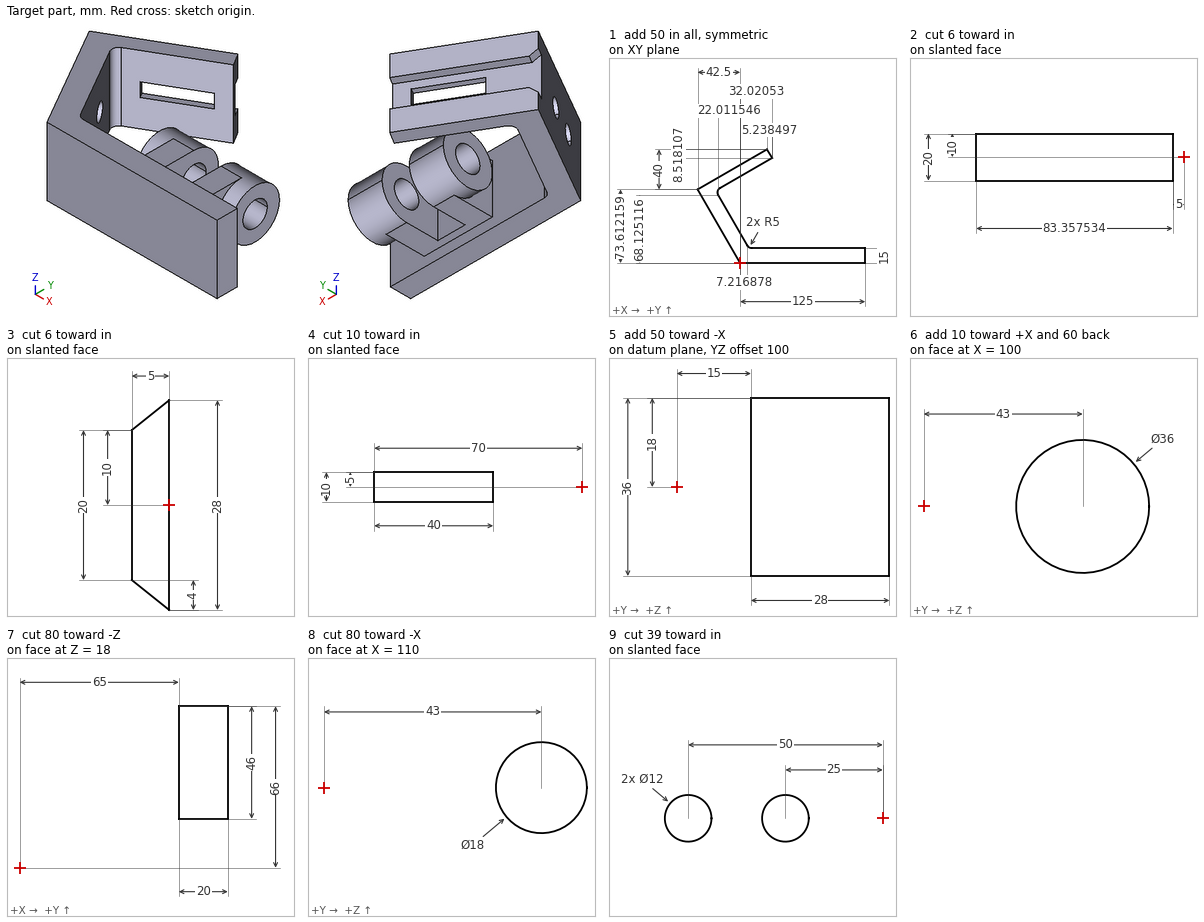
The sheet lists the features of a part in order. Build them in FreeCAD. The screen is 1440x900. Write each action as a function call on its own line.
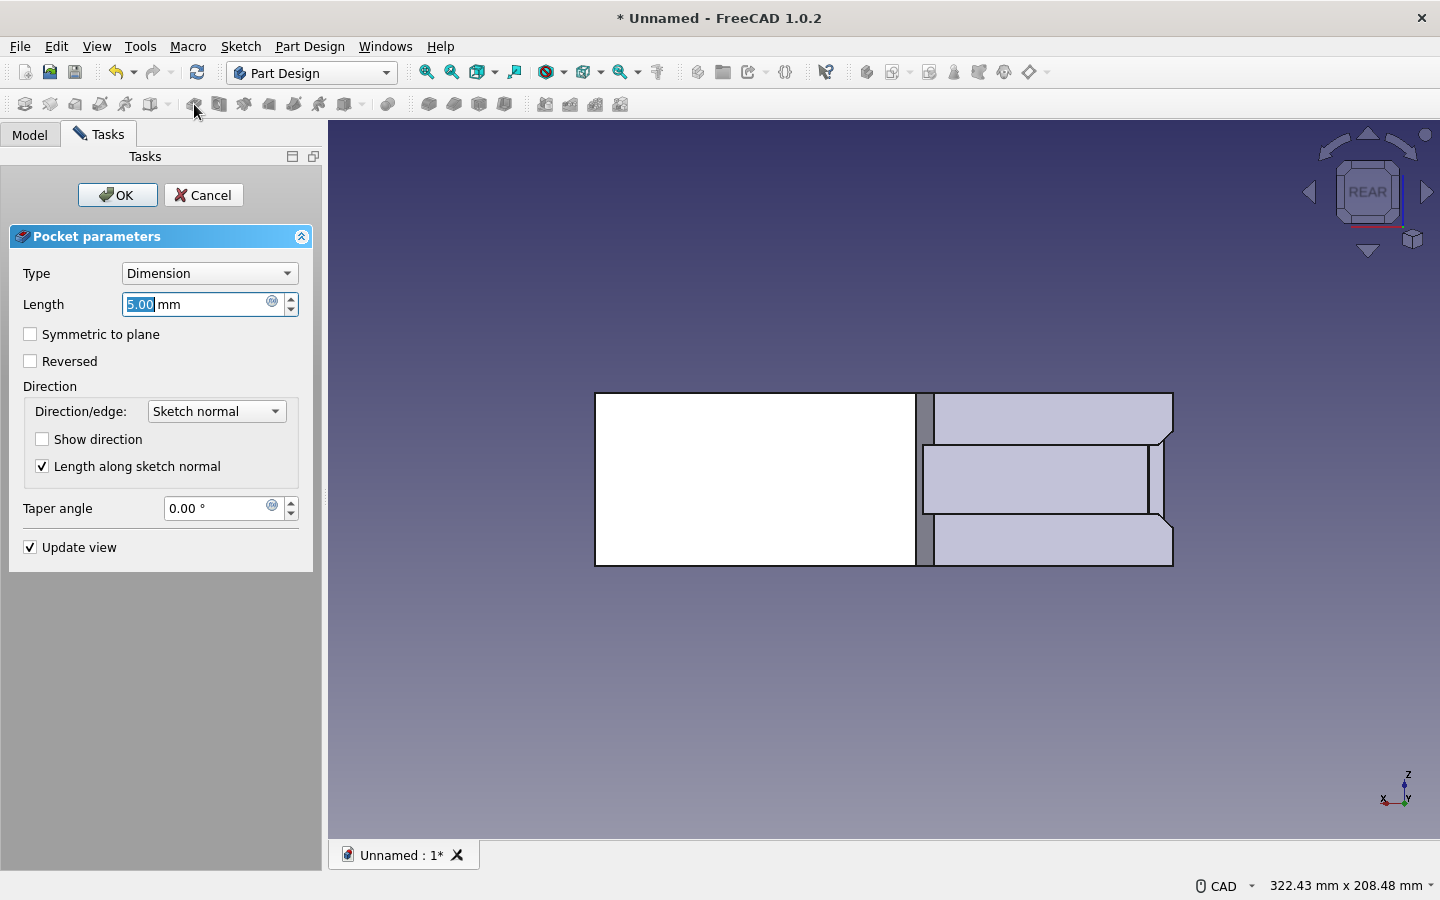
text(6)
key(Tab)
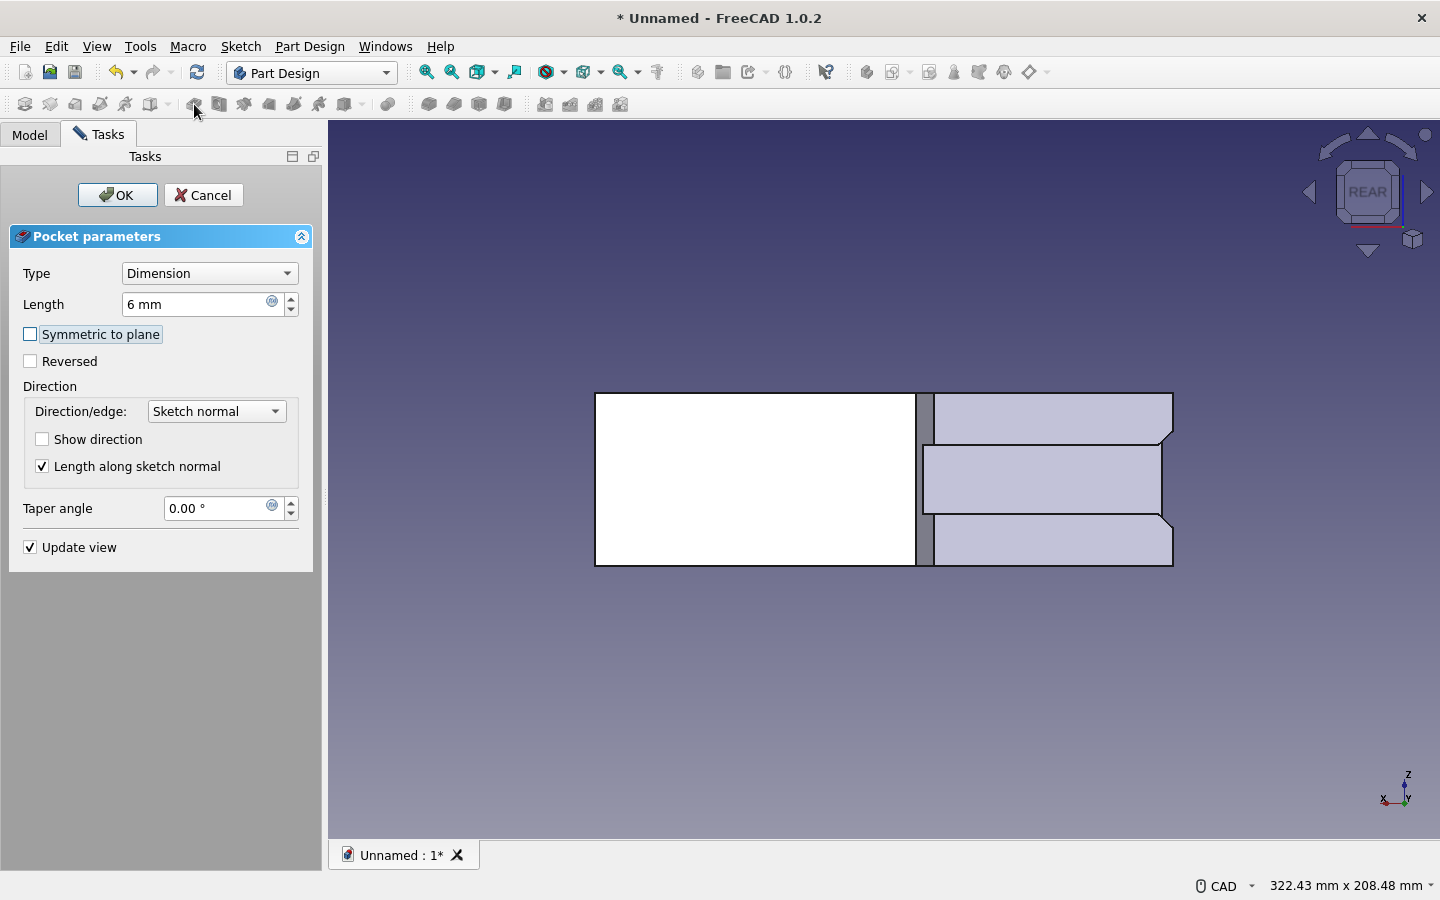
click(118, 195)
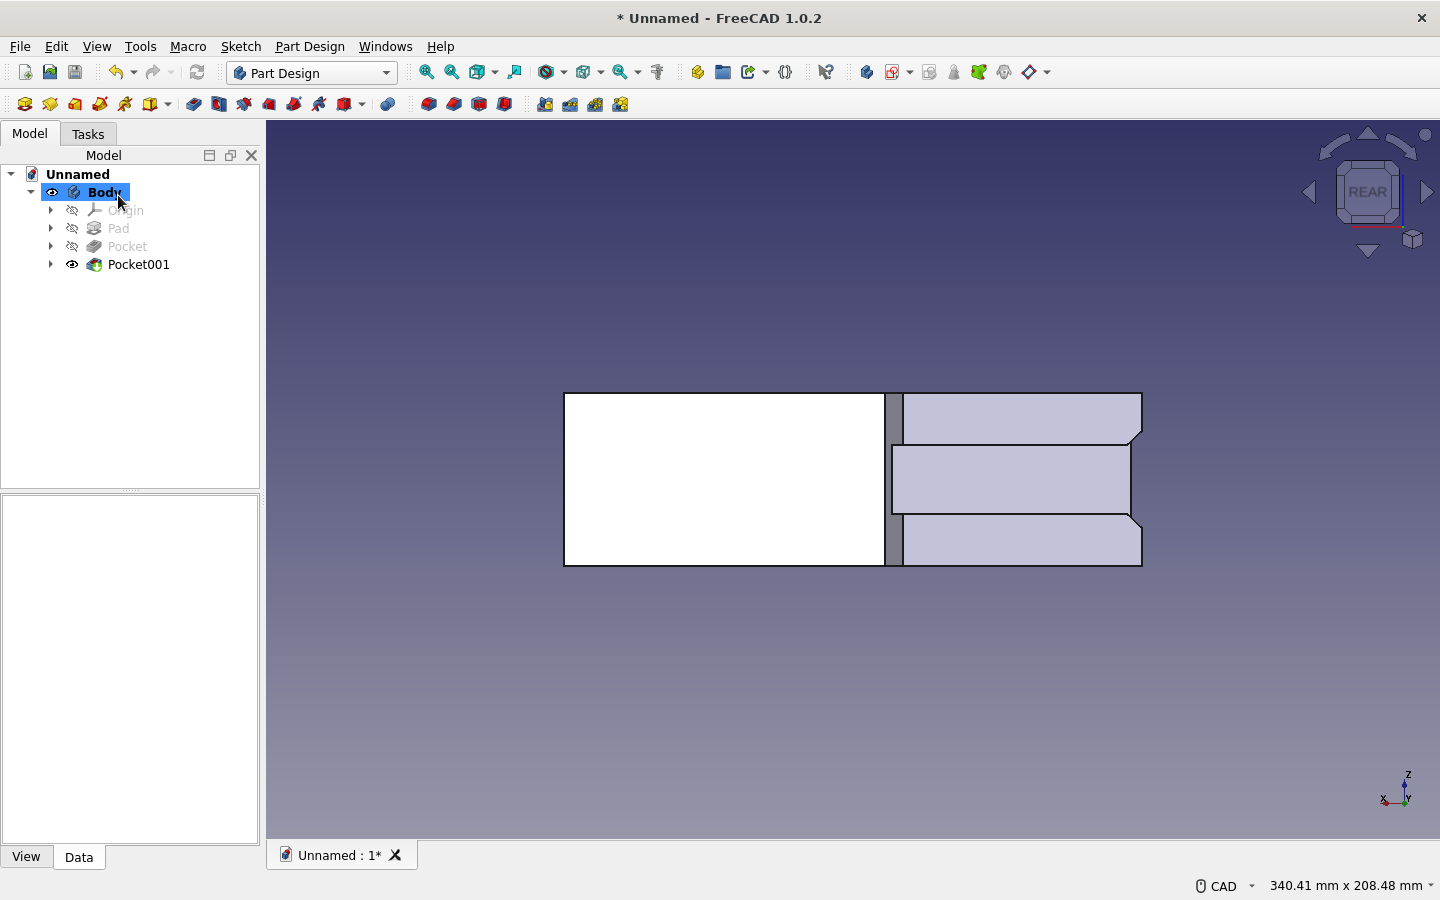
click(1046, 479)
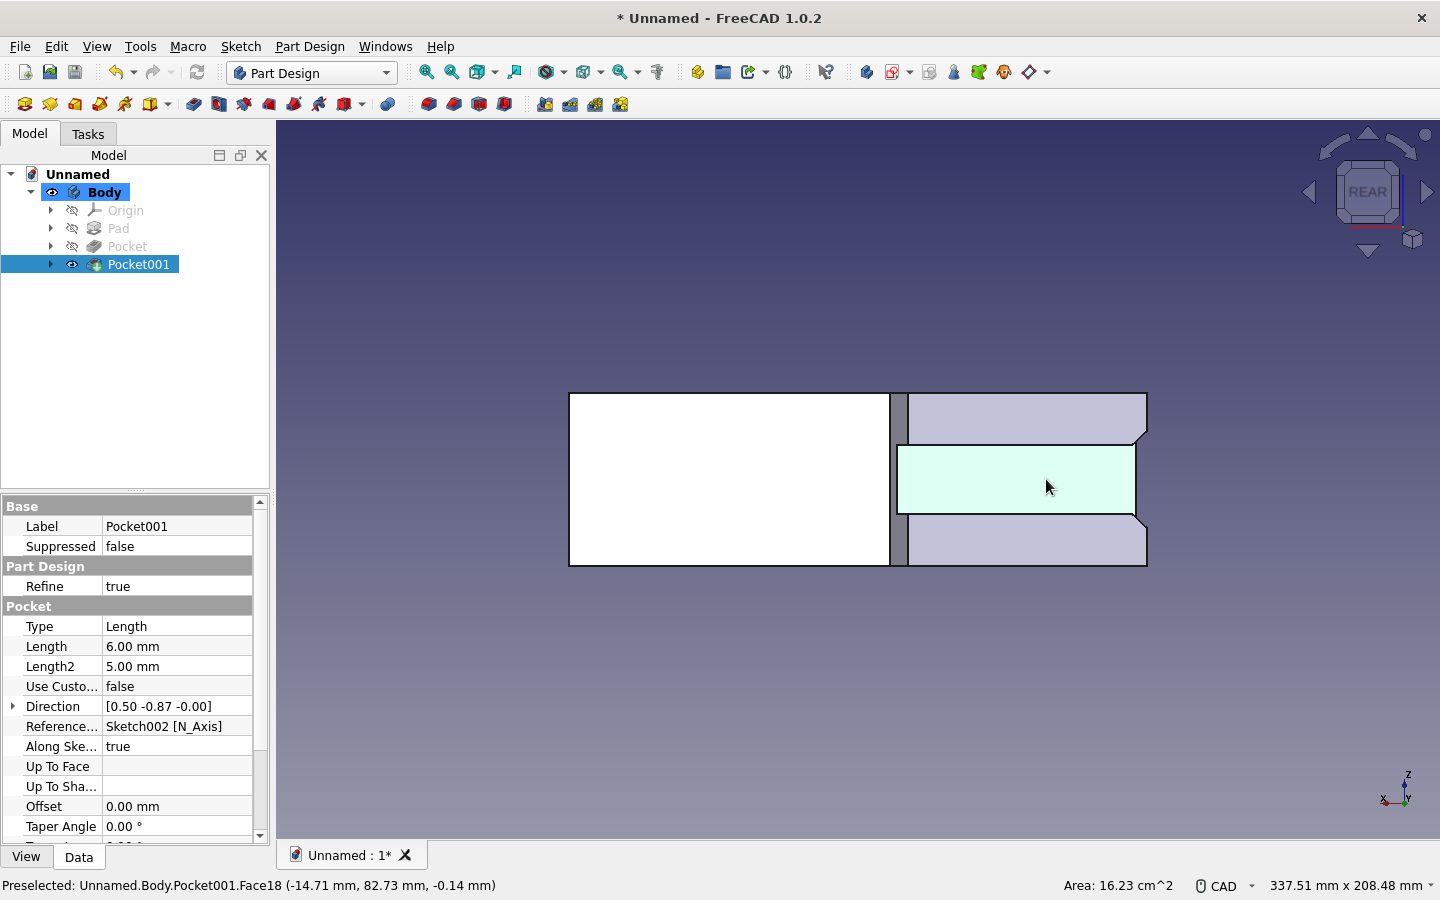
click(892, 72)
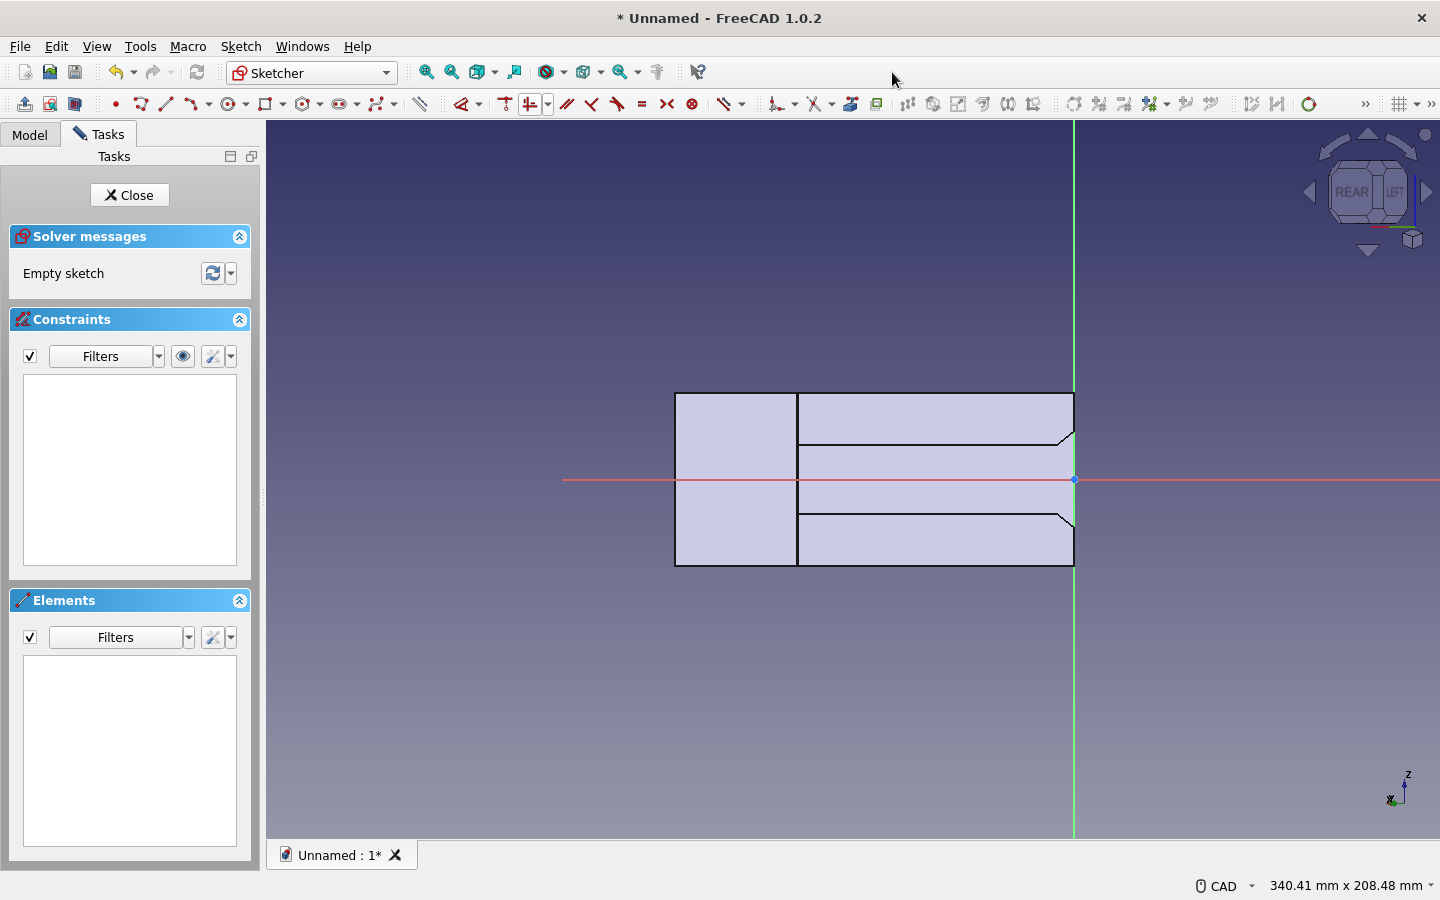
scroll(1052, 480, up, 5)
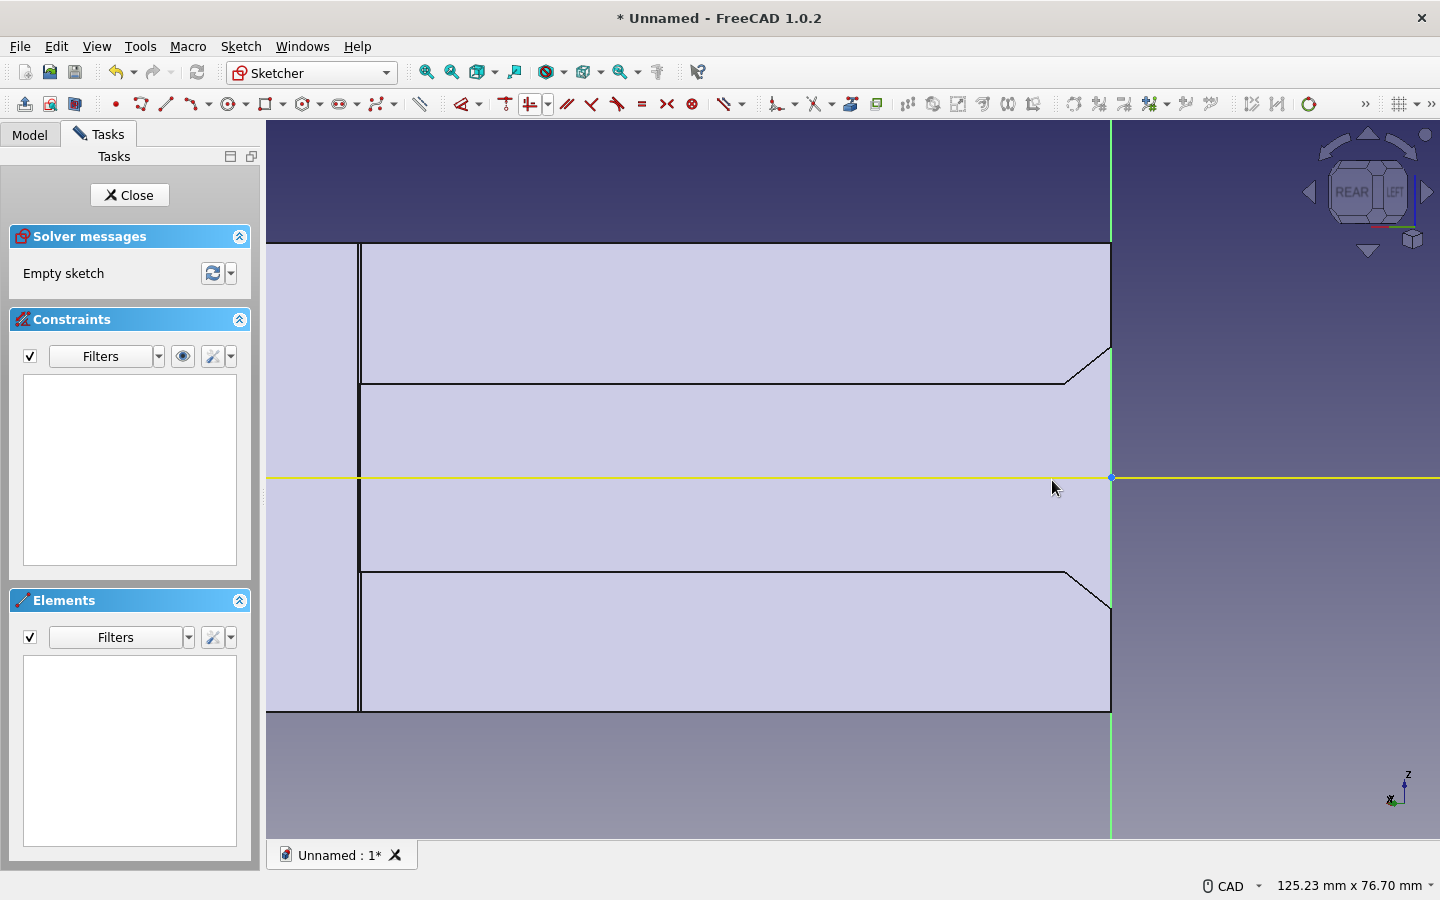
key(g)
key(r)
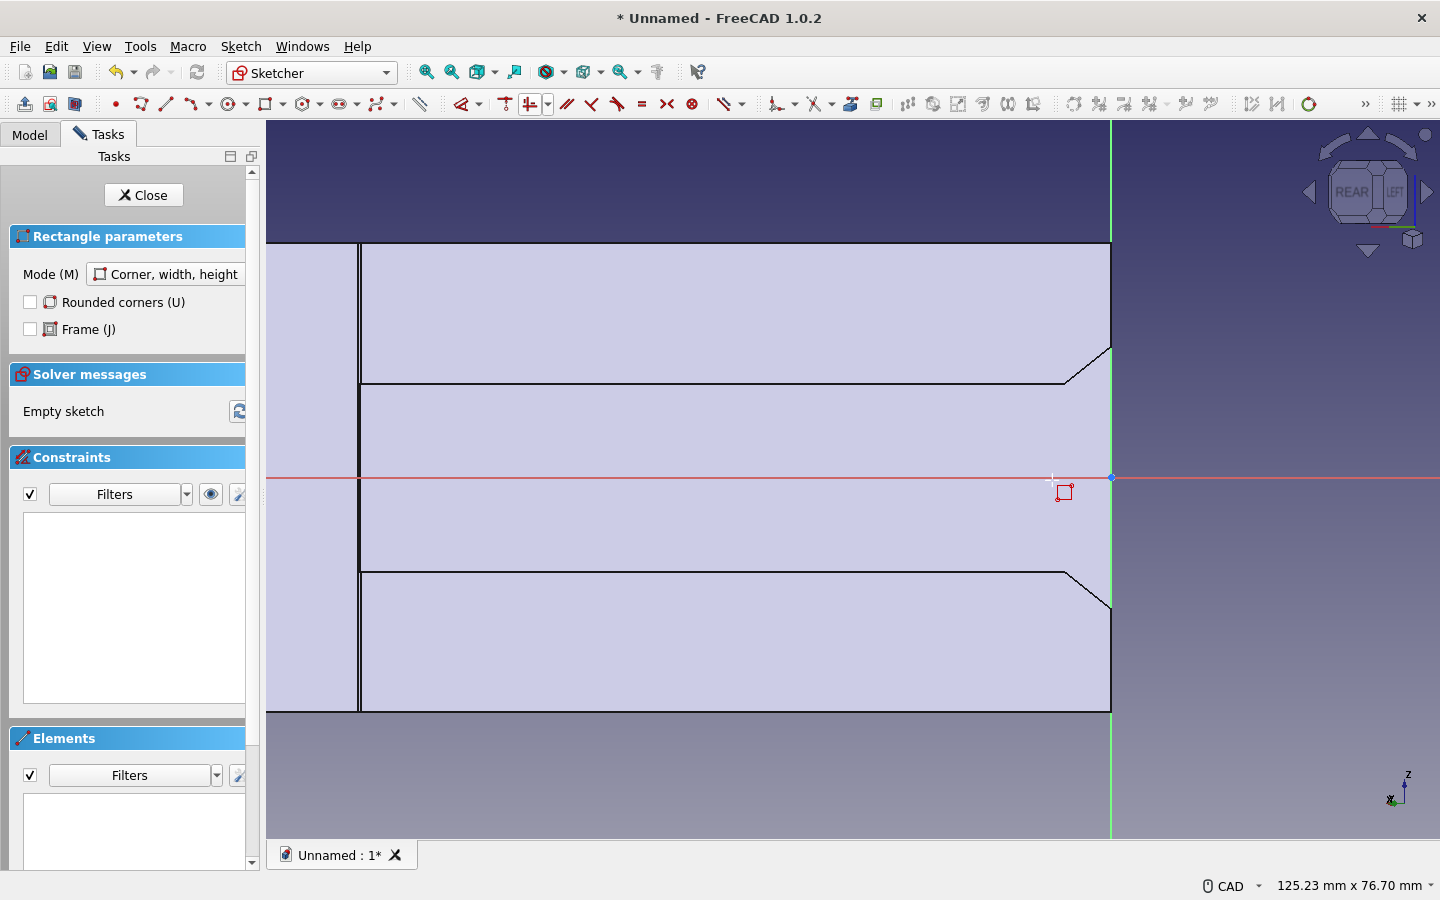
click(455, 431)
click(830, 525)
key(Escape)